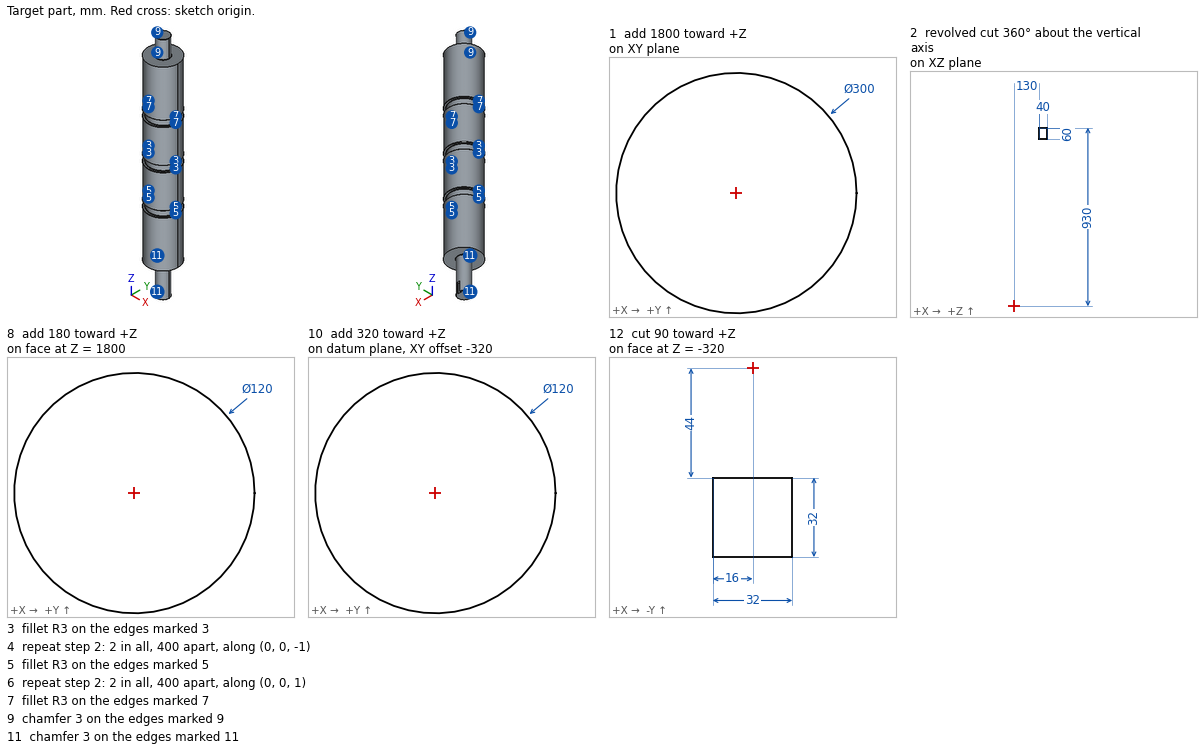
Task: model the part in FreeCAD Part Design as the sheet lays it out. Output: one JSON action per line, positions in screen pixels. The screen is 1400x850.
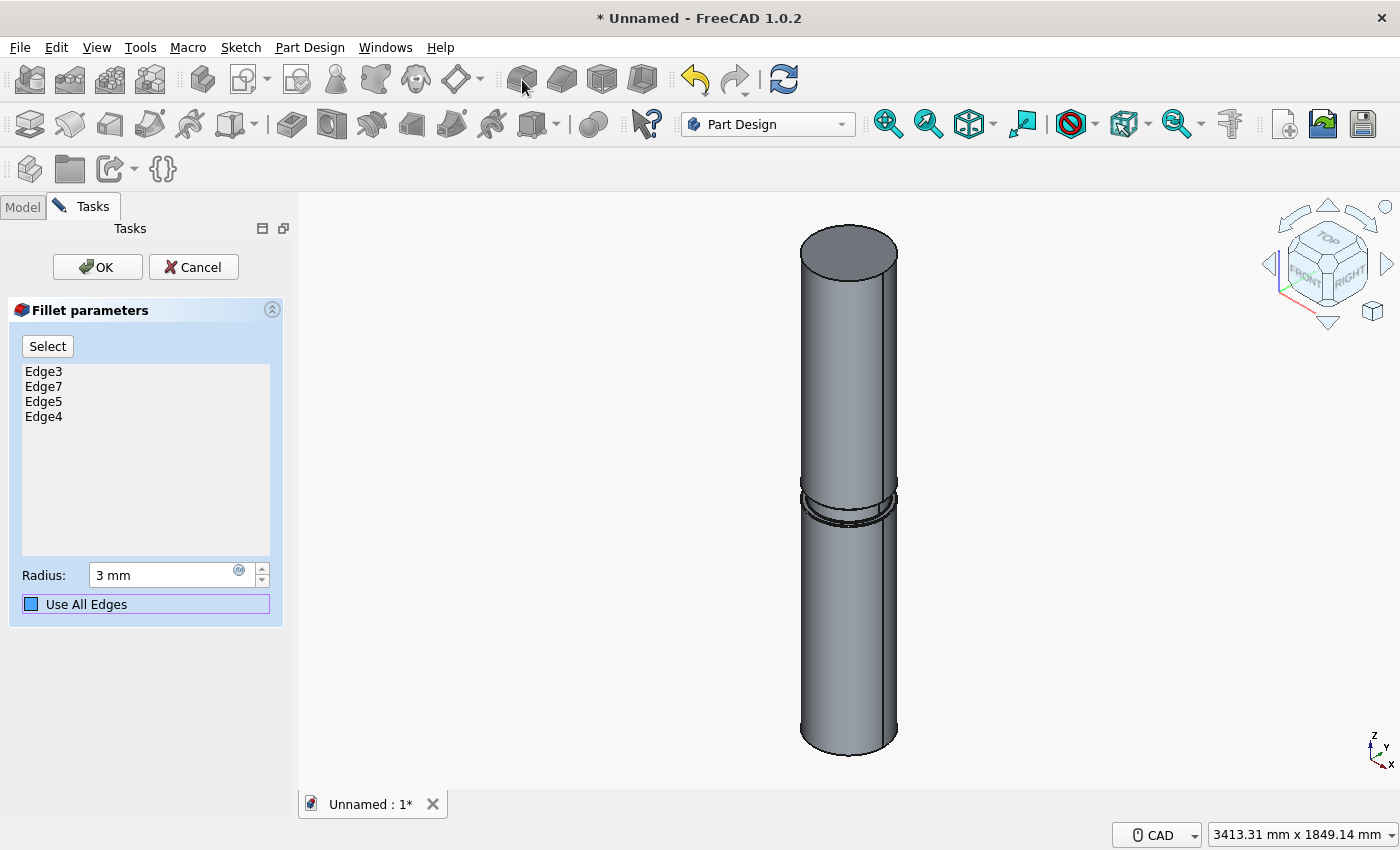
{"action": "left_click", "coordinate": [98, 267]}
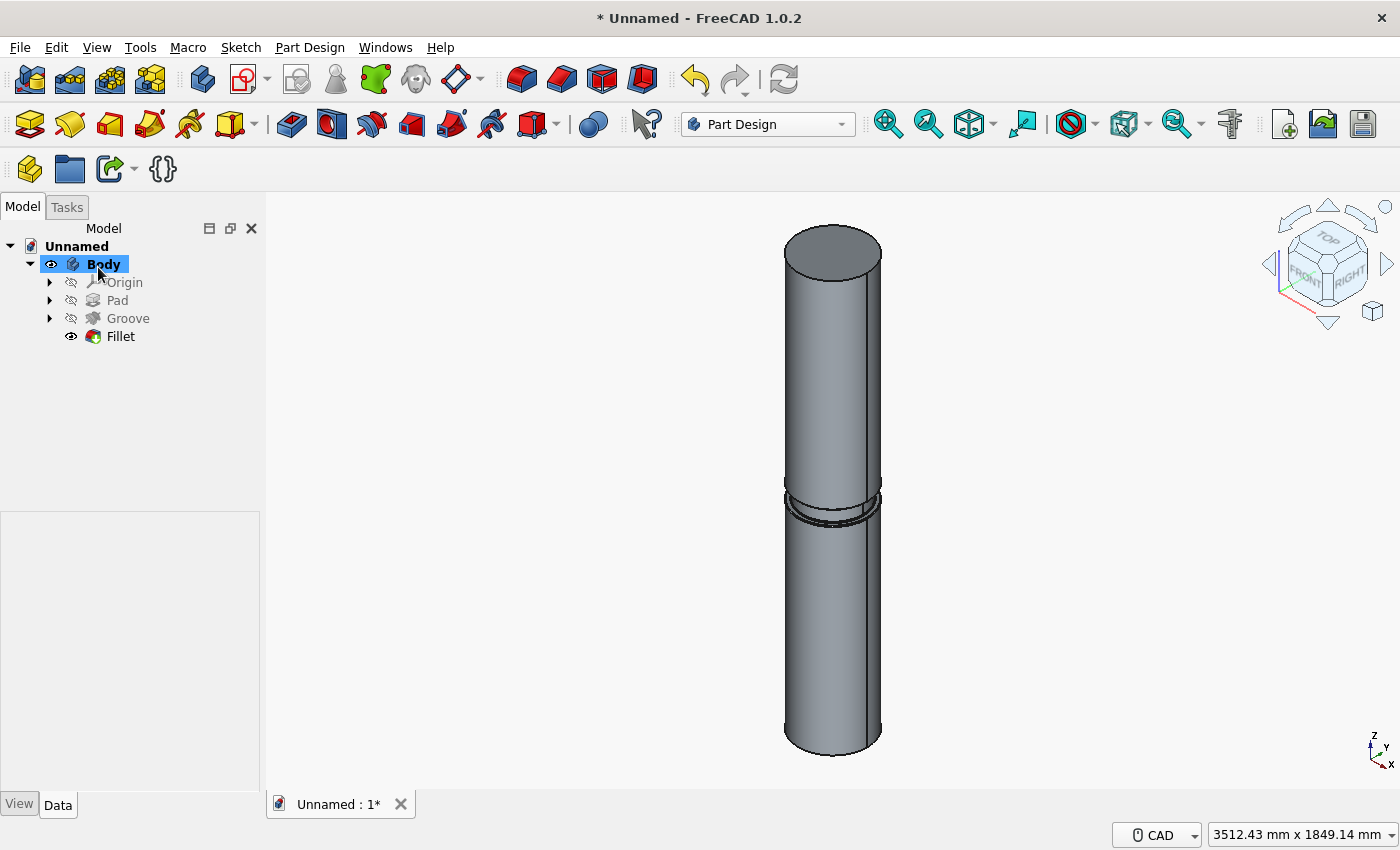
{"action": "left_click", "coordinate": [116, 318]}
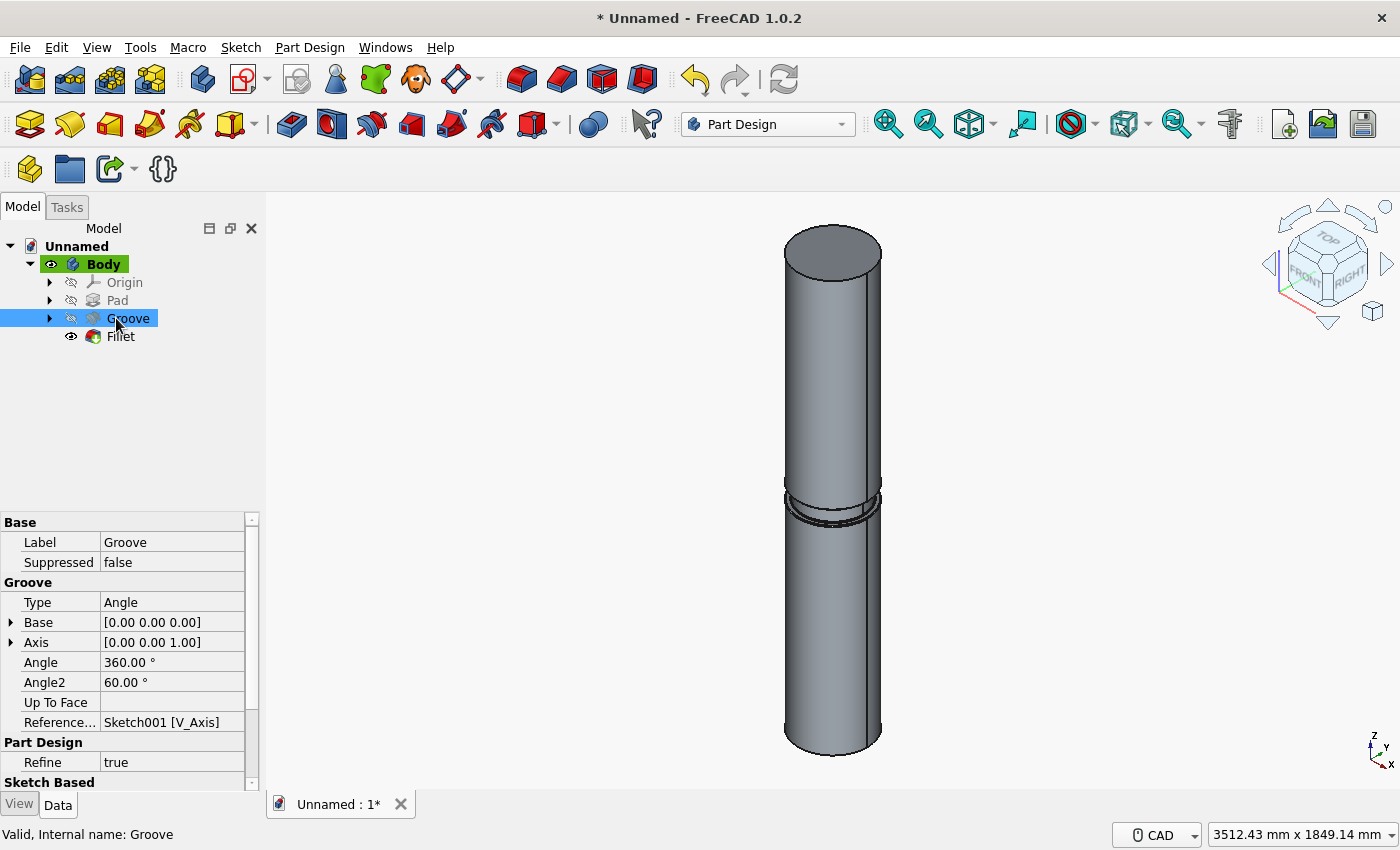
{"action": "left_click", "coordinate": [70, 80]}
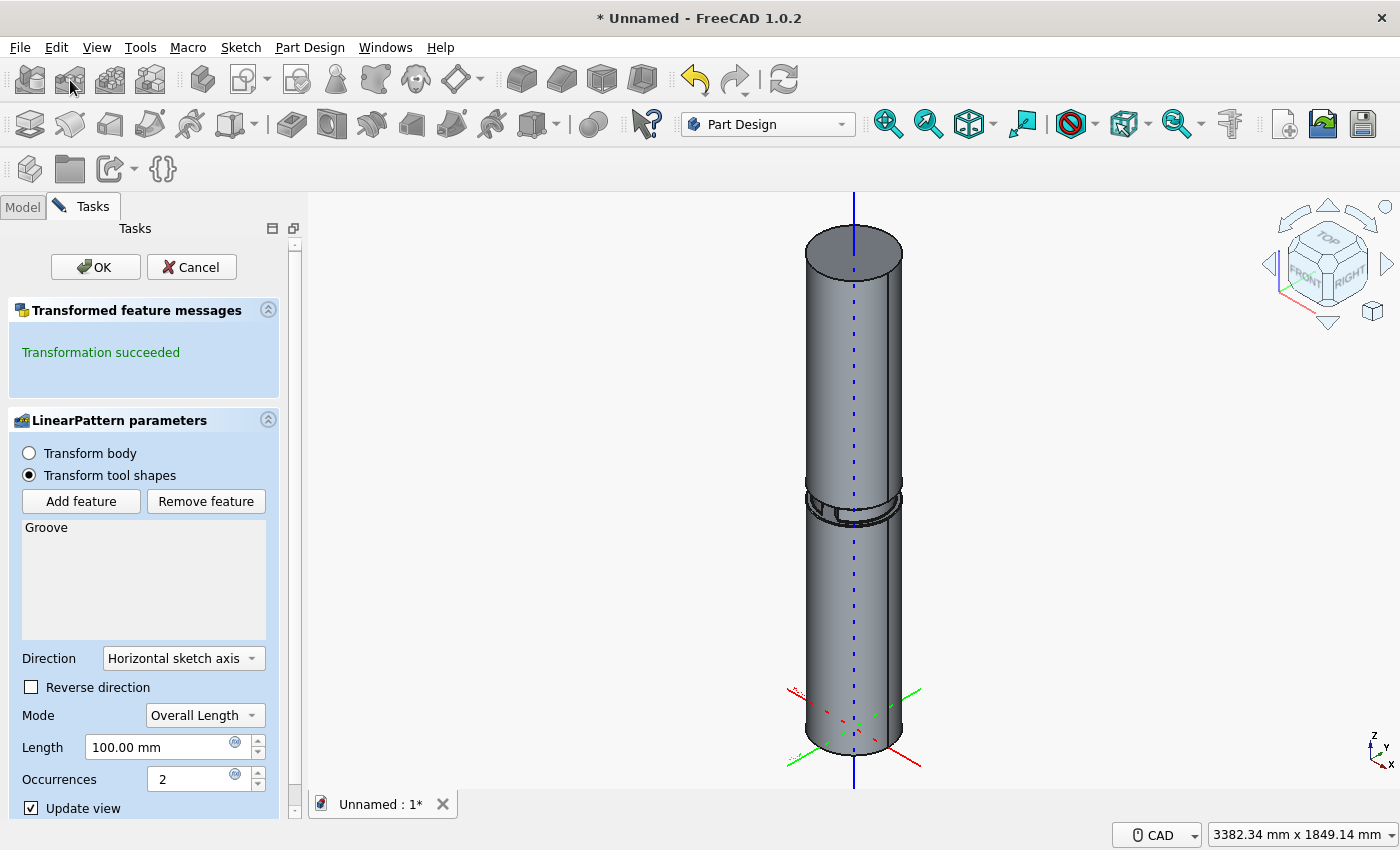
{"action": "left_click", "coordinate": [184, 658]}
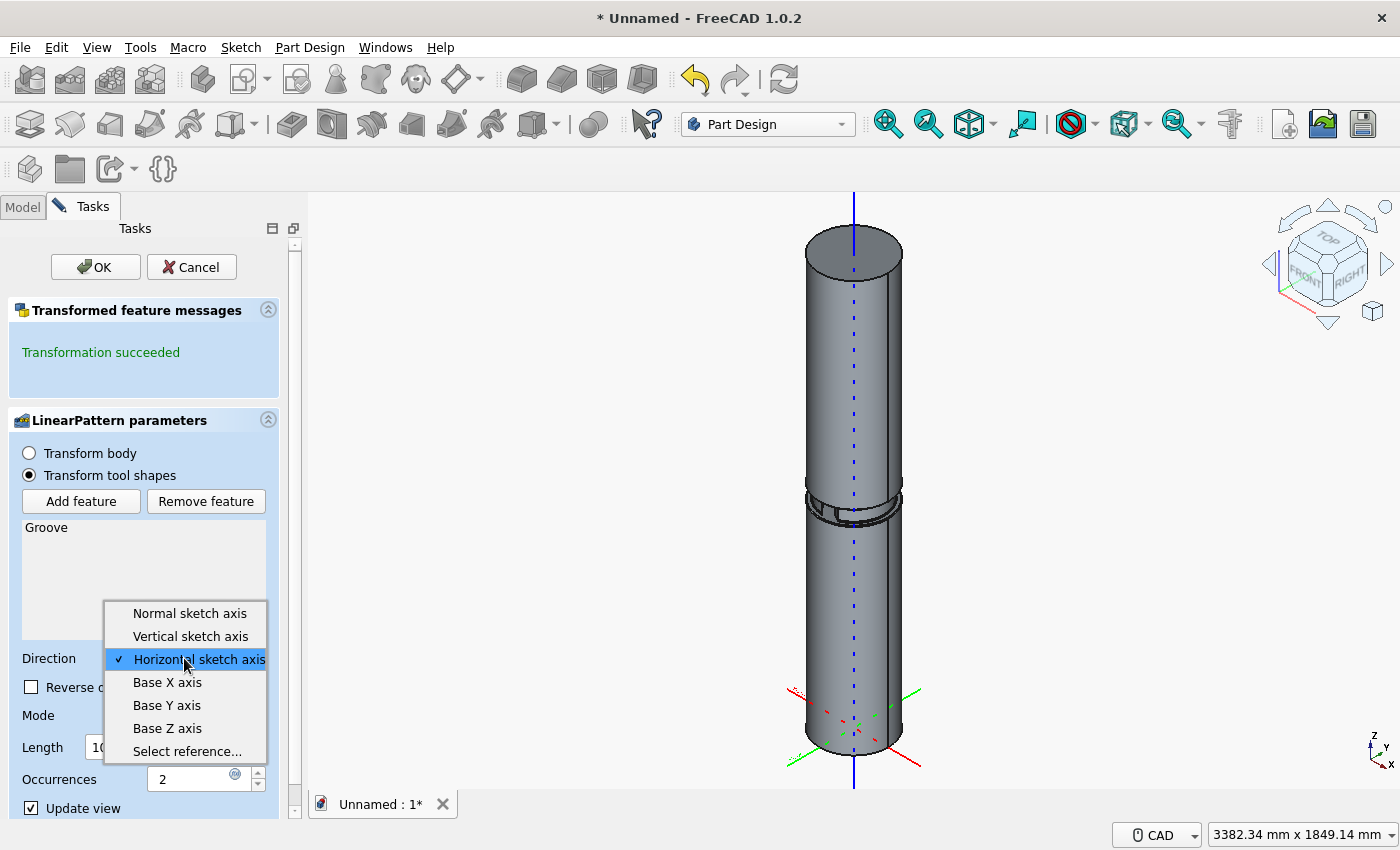
{"action": "left_click", "coordinate": [184, 728]}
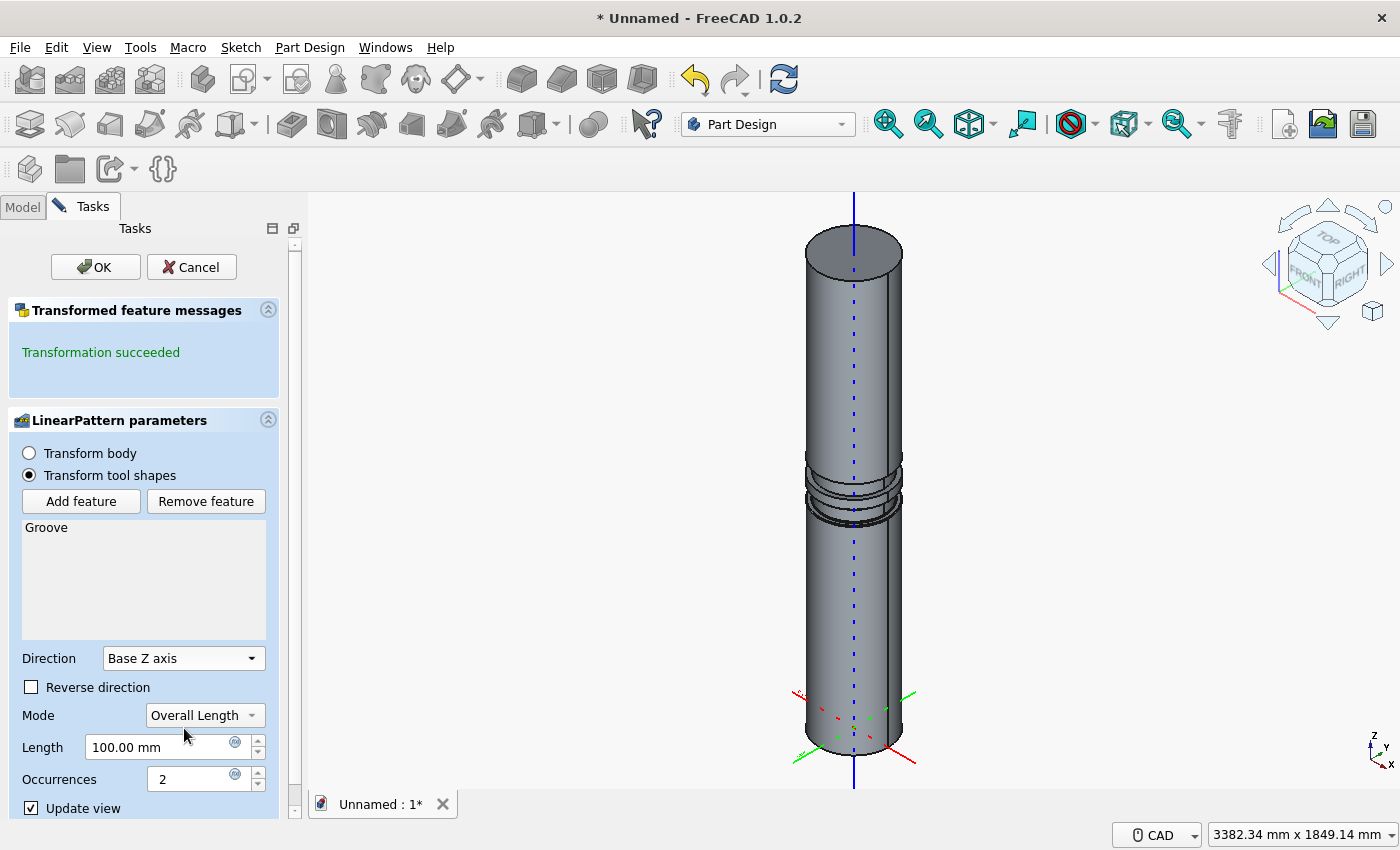
{"action": "left_click", "coordinate": [206, 716]}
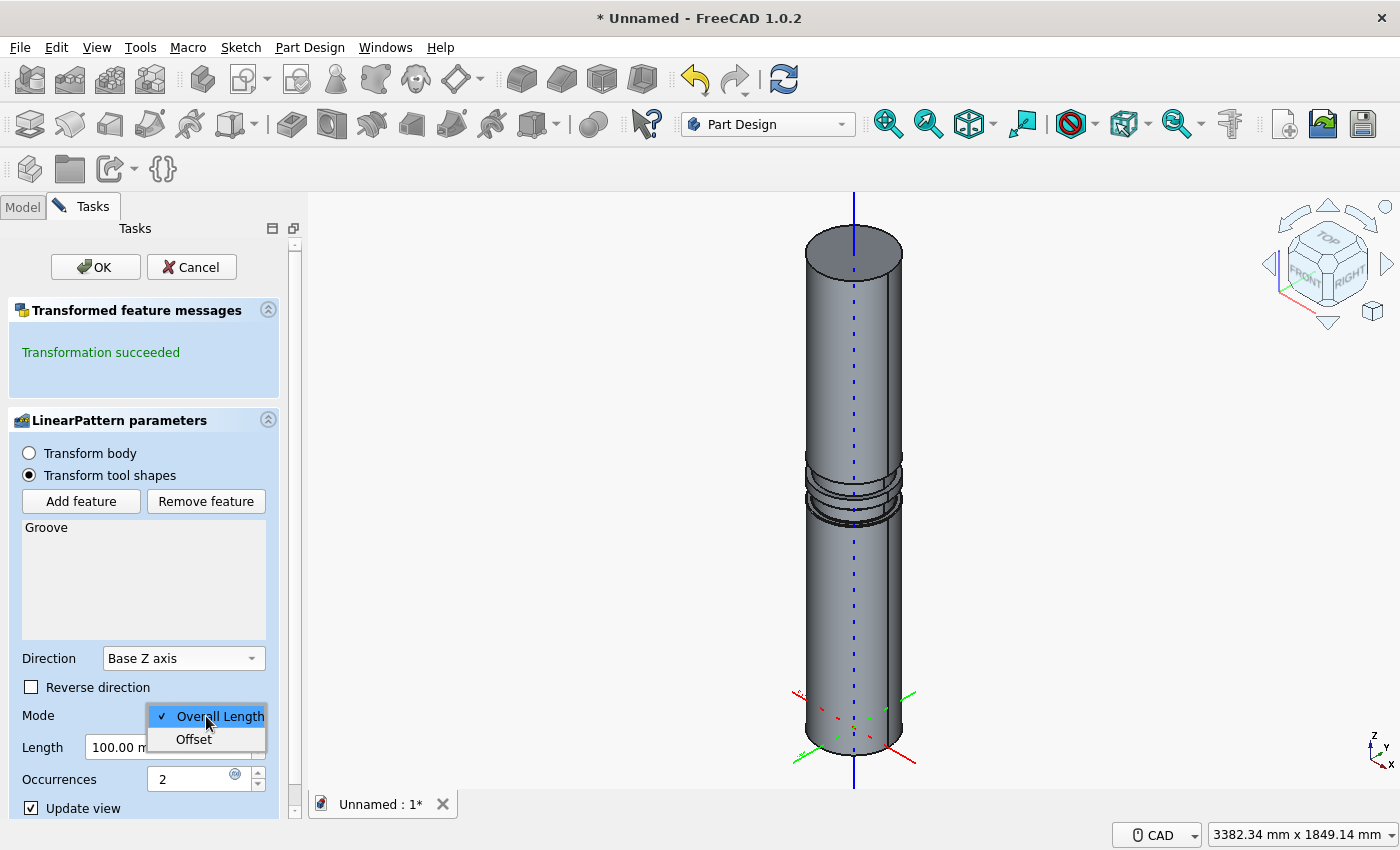
{"action": "left_click", "coordinate": [206, 740]}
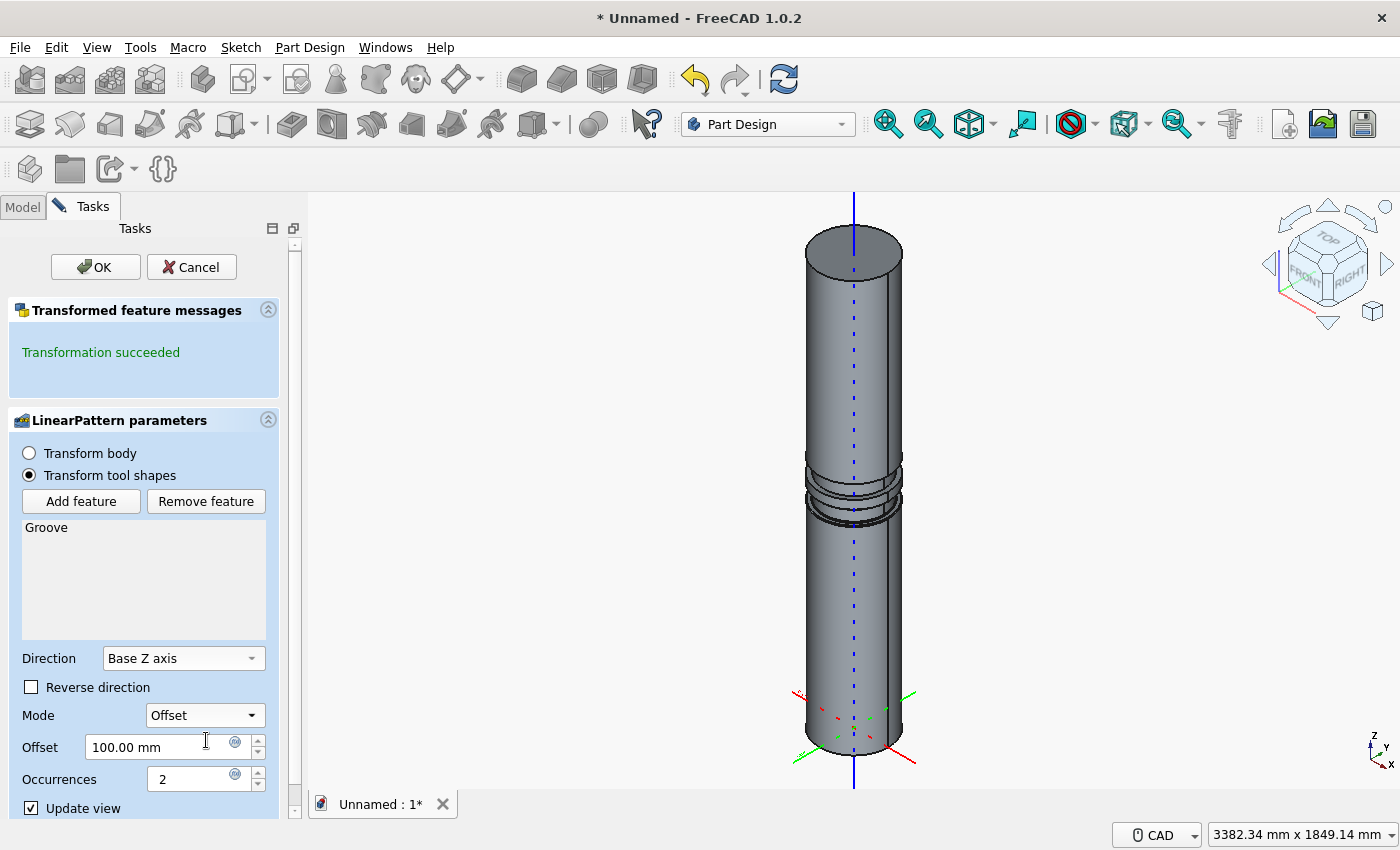
{"action": "triple_click", "coordinate": [168, 747]}